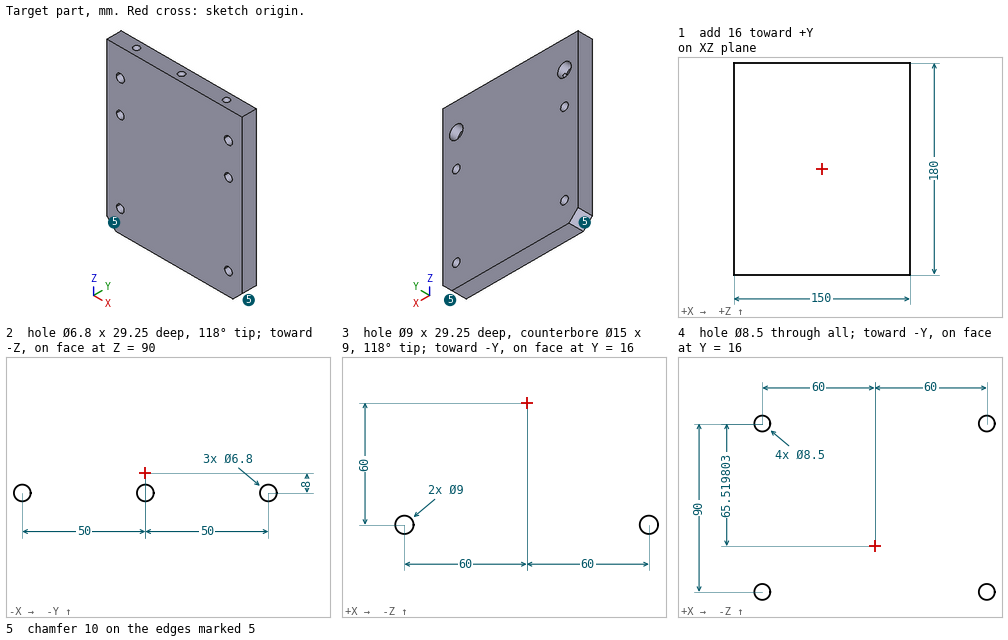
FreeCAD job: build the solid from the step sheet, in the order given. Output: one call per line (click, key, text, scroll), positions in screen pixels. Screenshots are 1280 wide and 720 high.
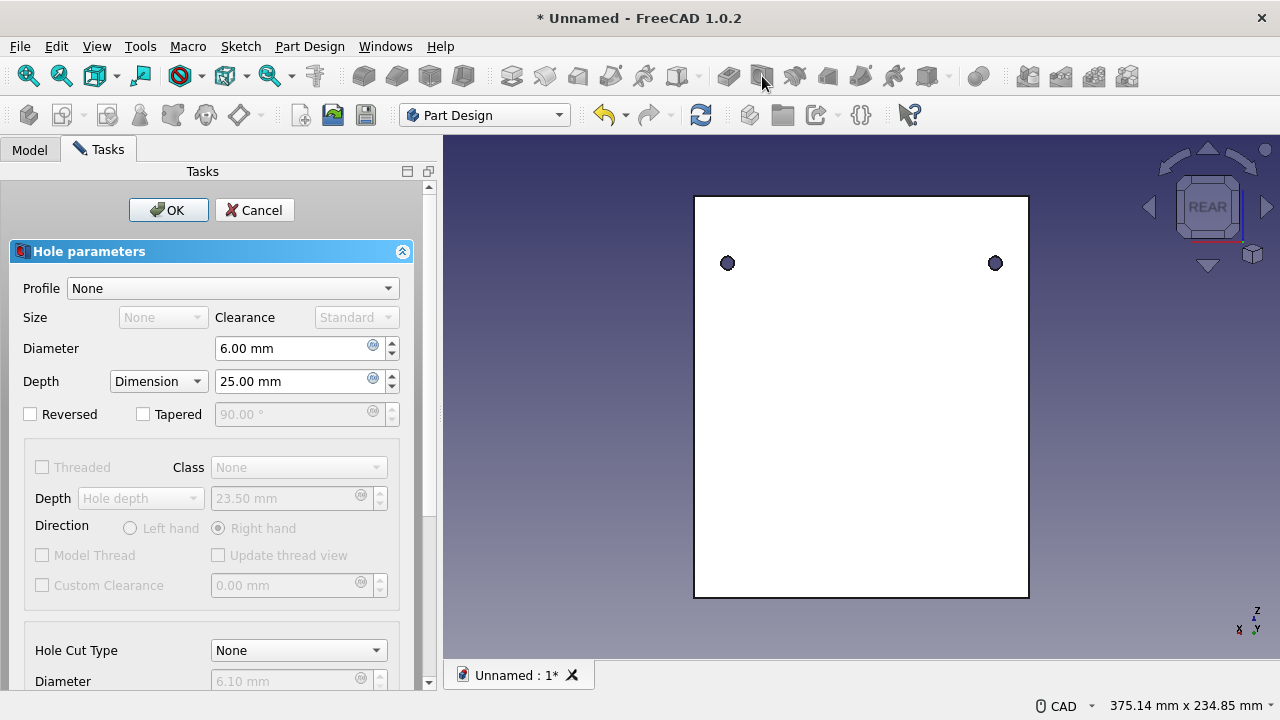
triple_click(300, 348)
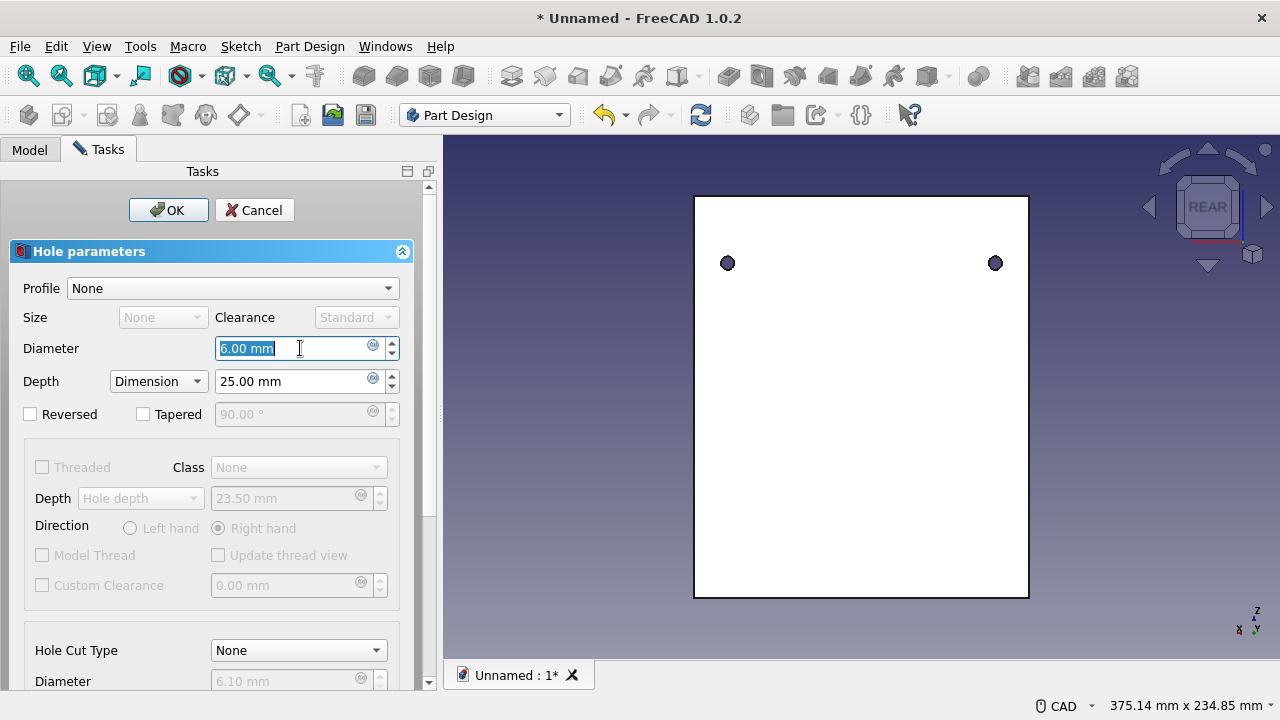
text(9)
key(Tab)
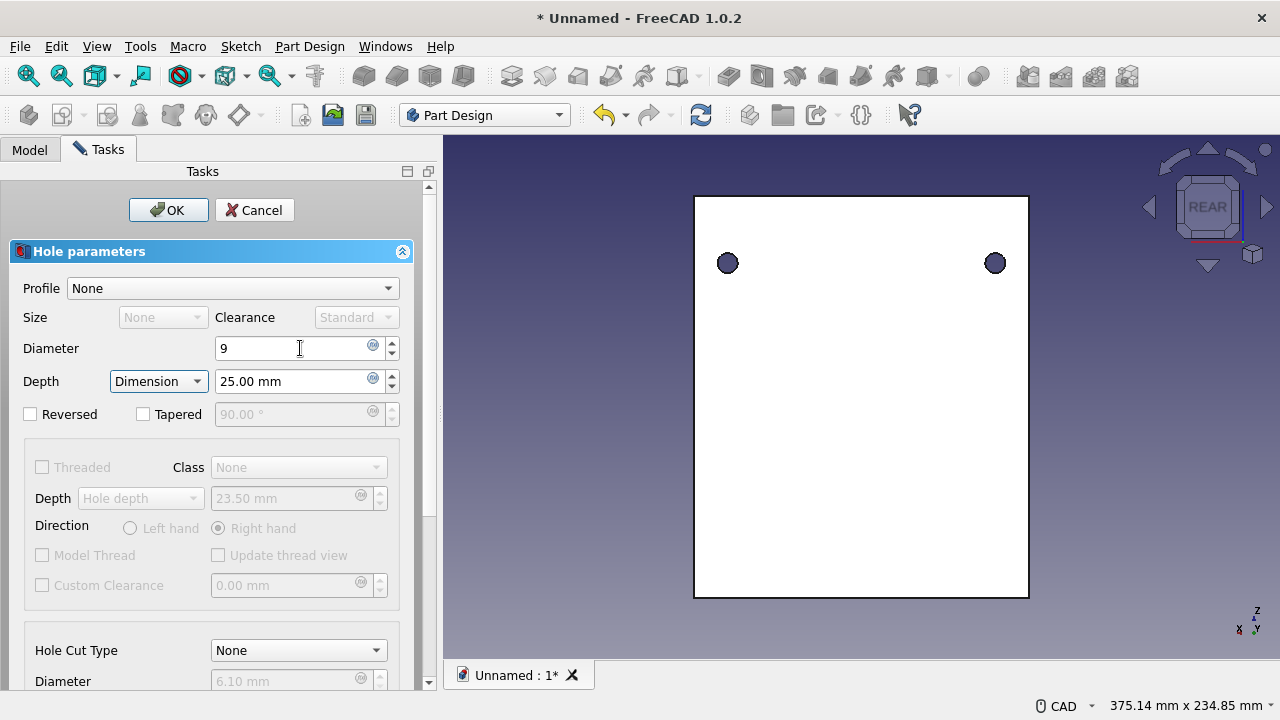
triple_click(300, 382)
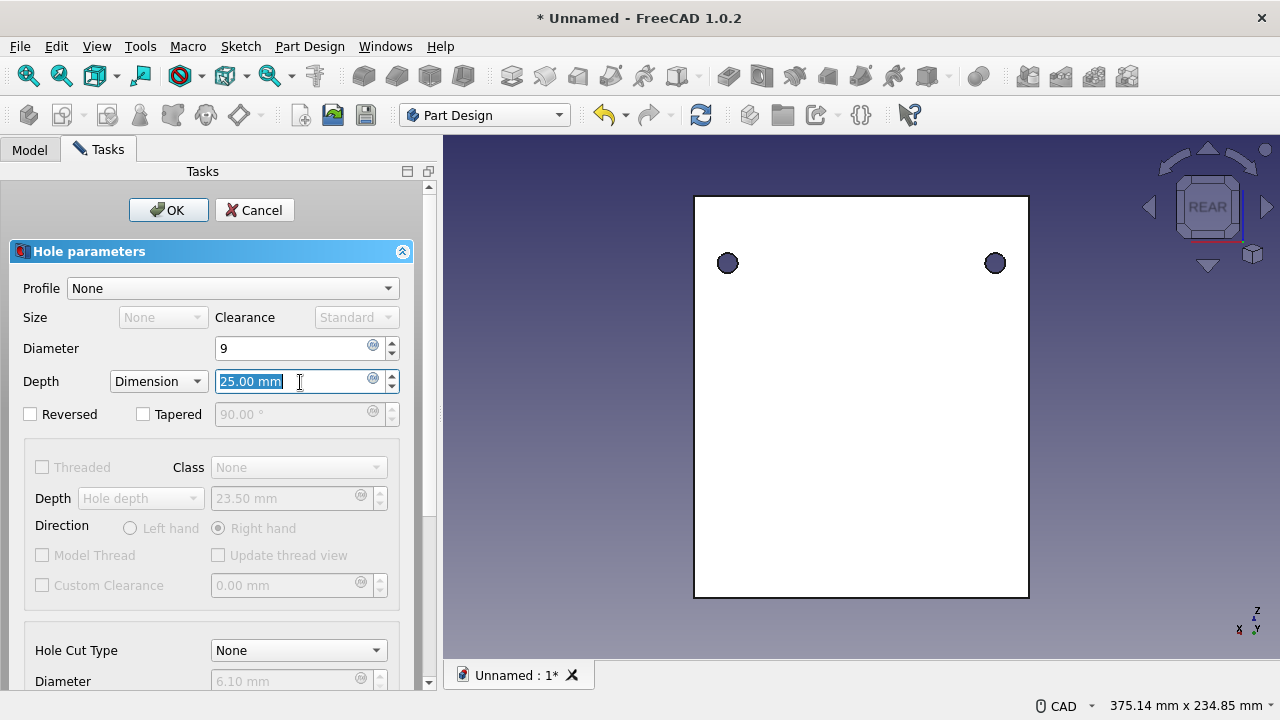
text(29.25)
key(Tab)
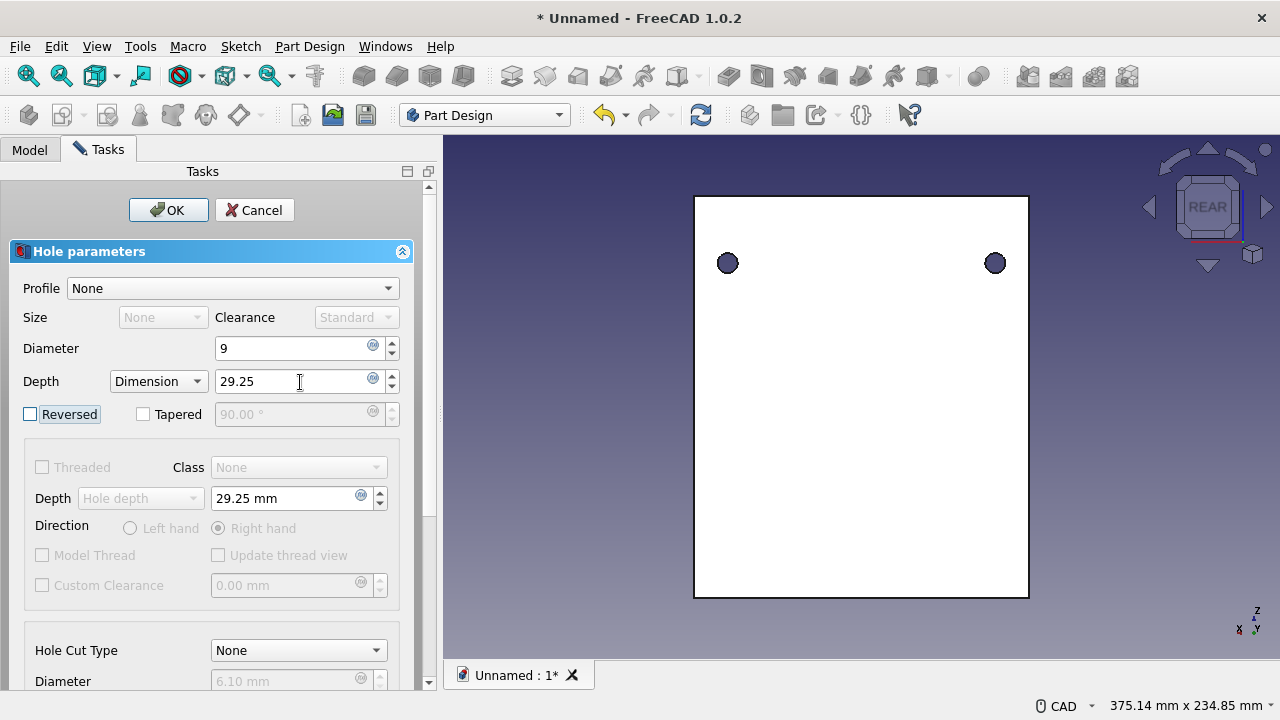
click(300, 650)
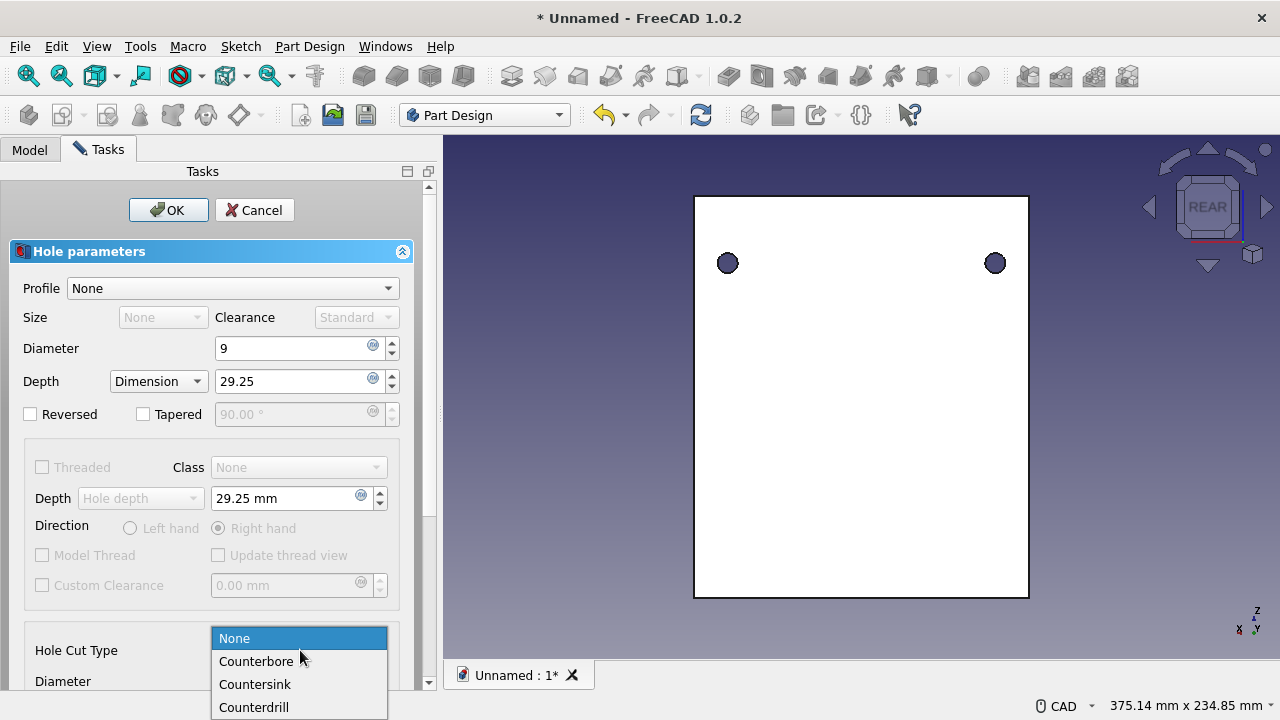
click(298, 662)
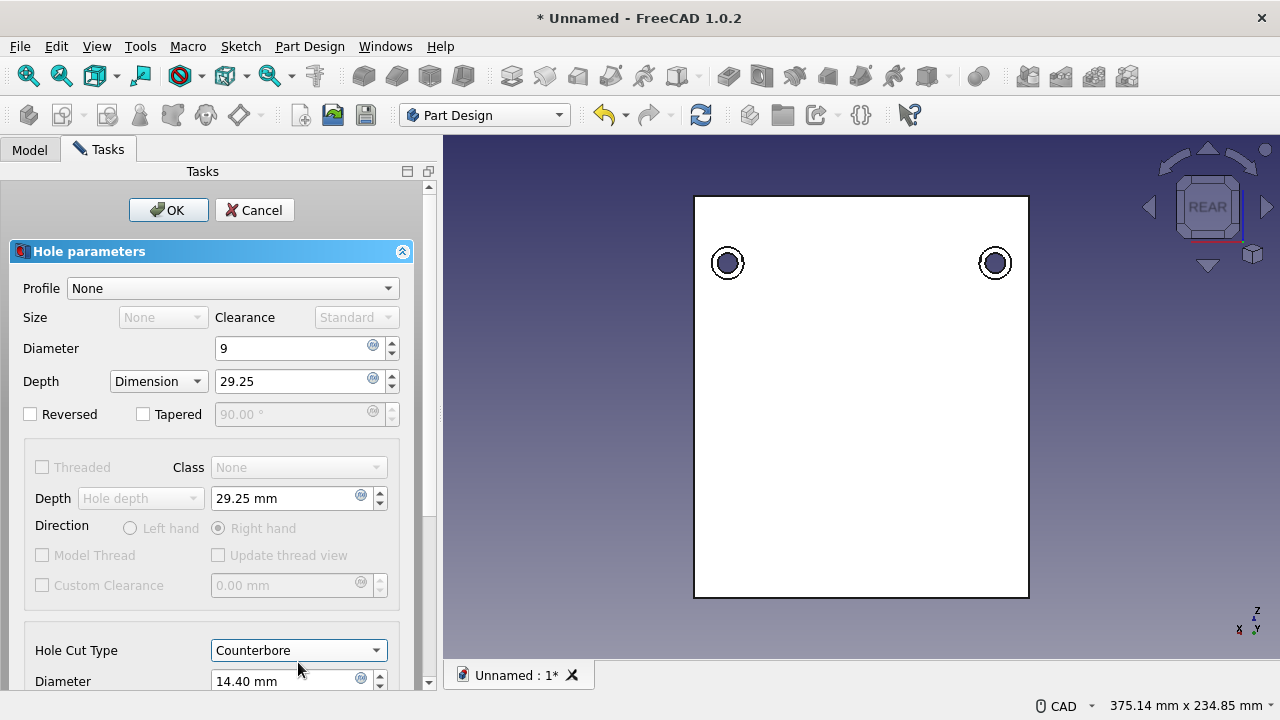
scroll(429, 436, down, 2)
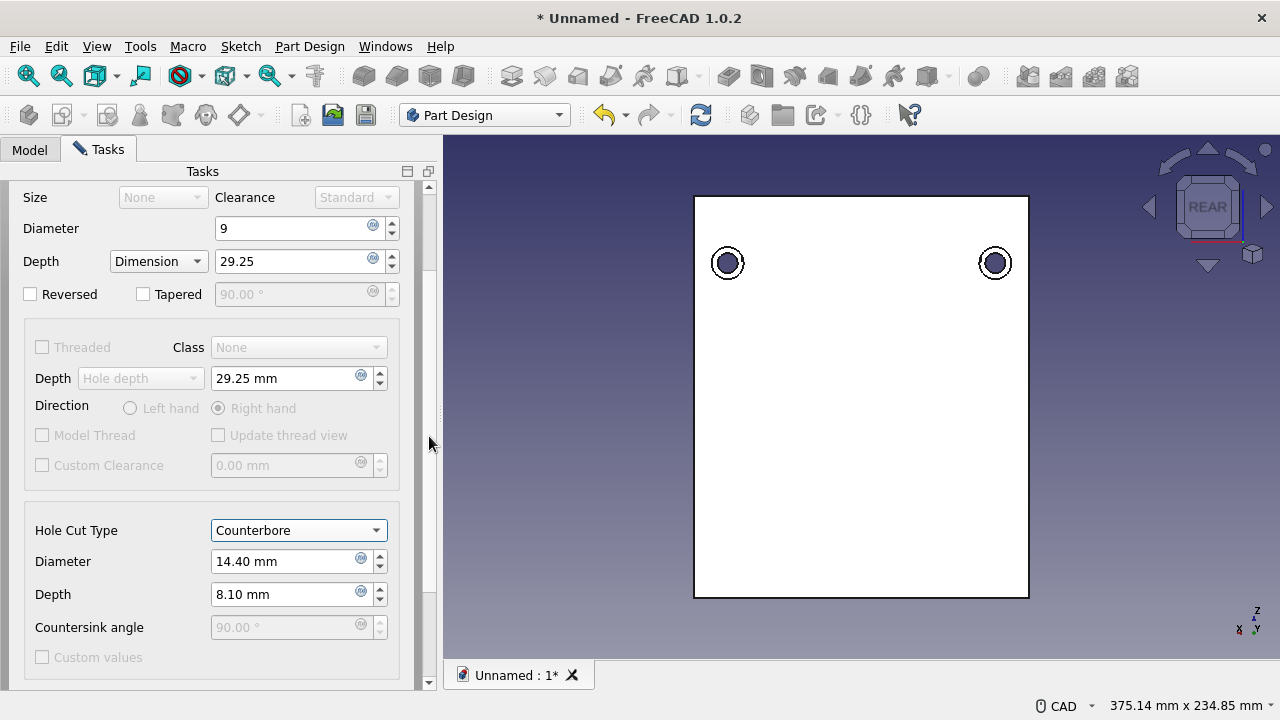
triple_click(292, 562)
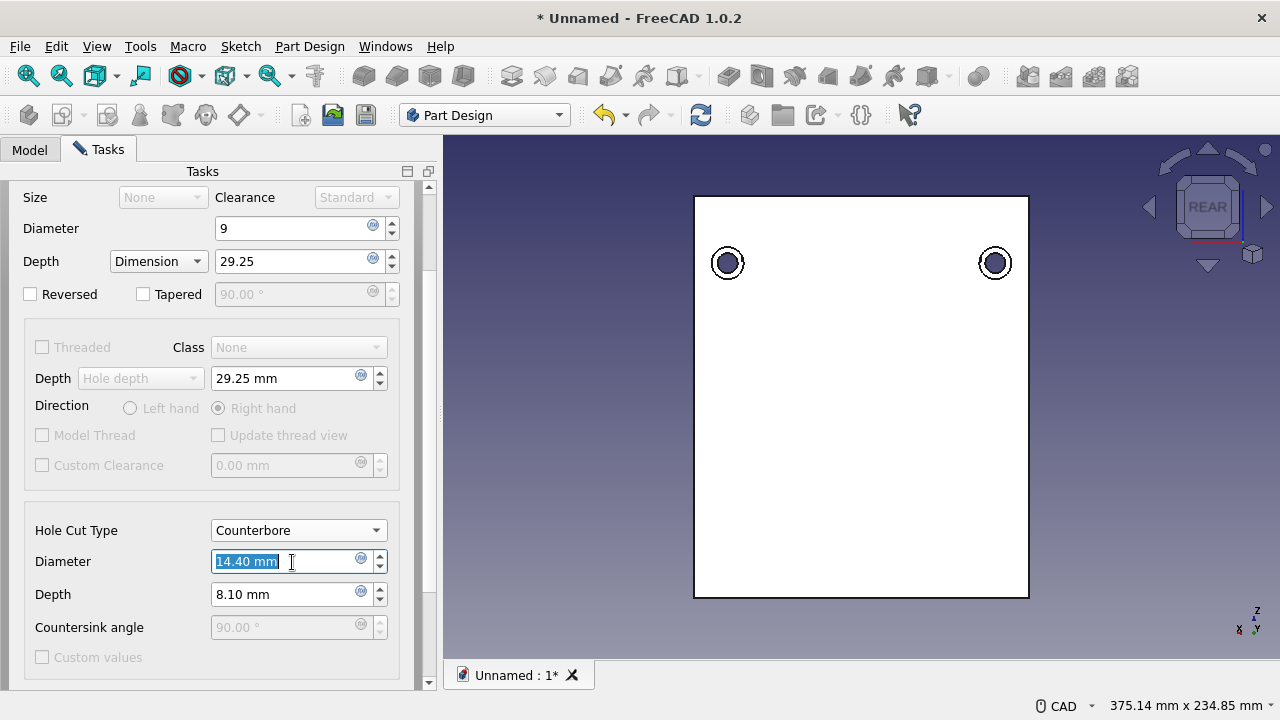
text(15)
key(Tab)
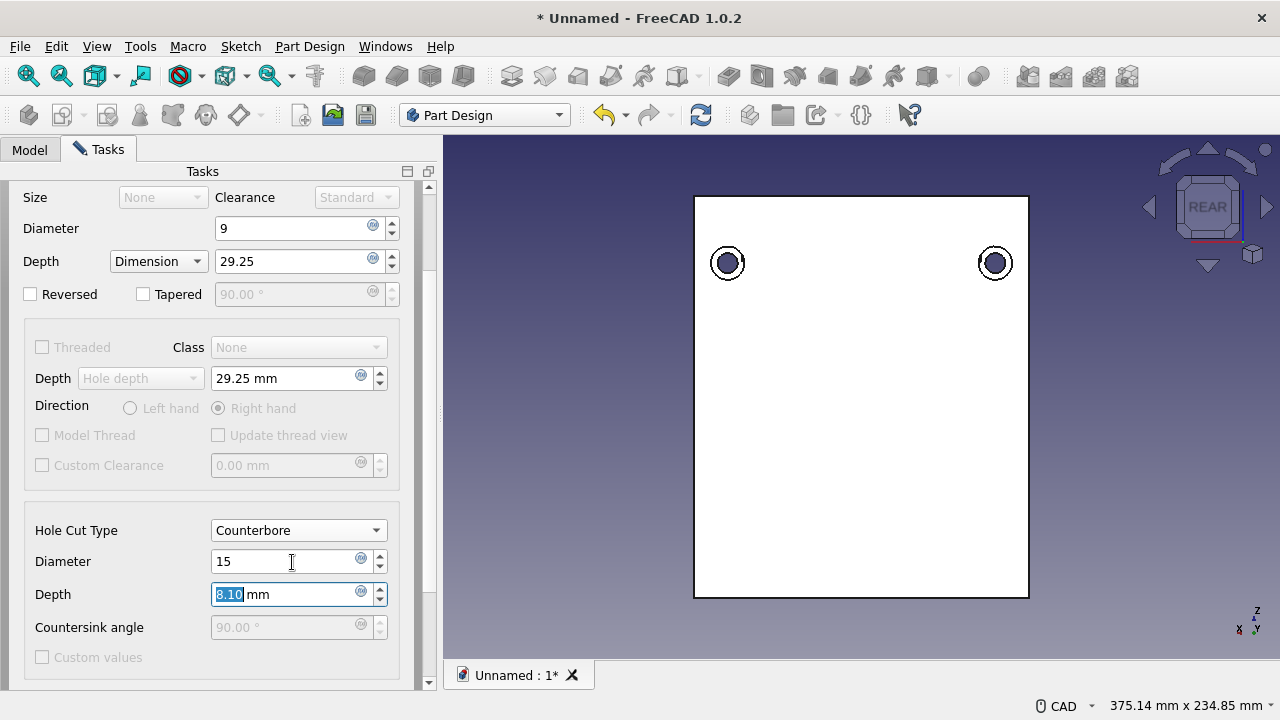
text(9)
key(Tab)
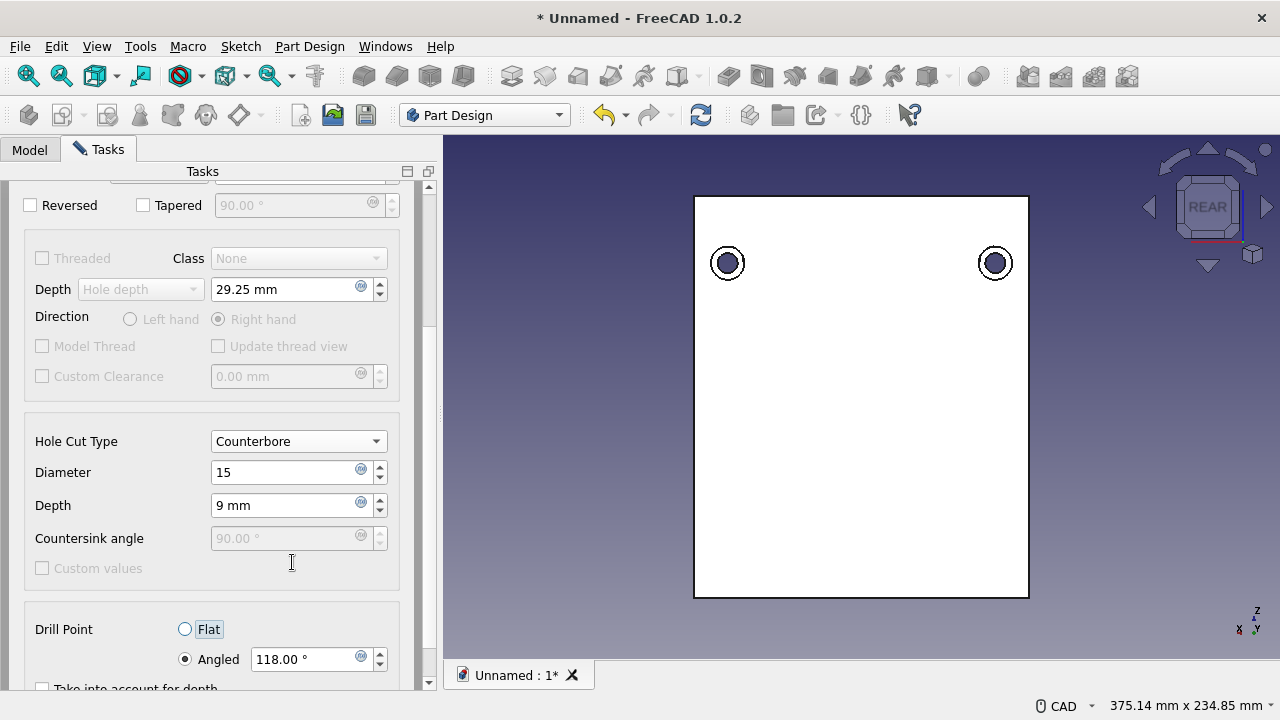
scroll(429, 436, up, 5)